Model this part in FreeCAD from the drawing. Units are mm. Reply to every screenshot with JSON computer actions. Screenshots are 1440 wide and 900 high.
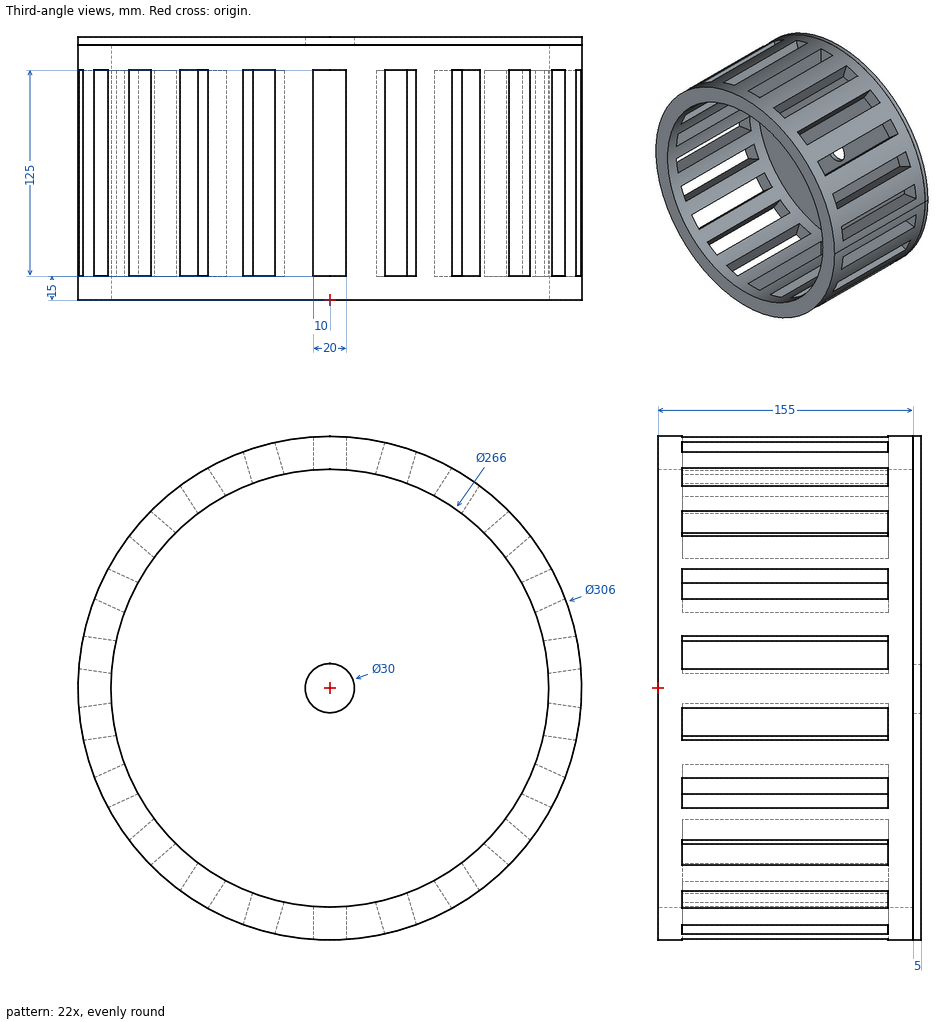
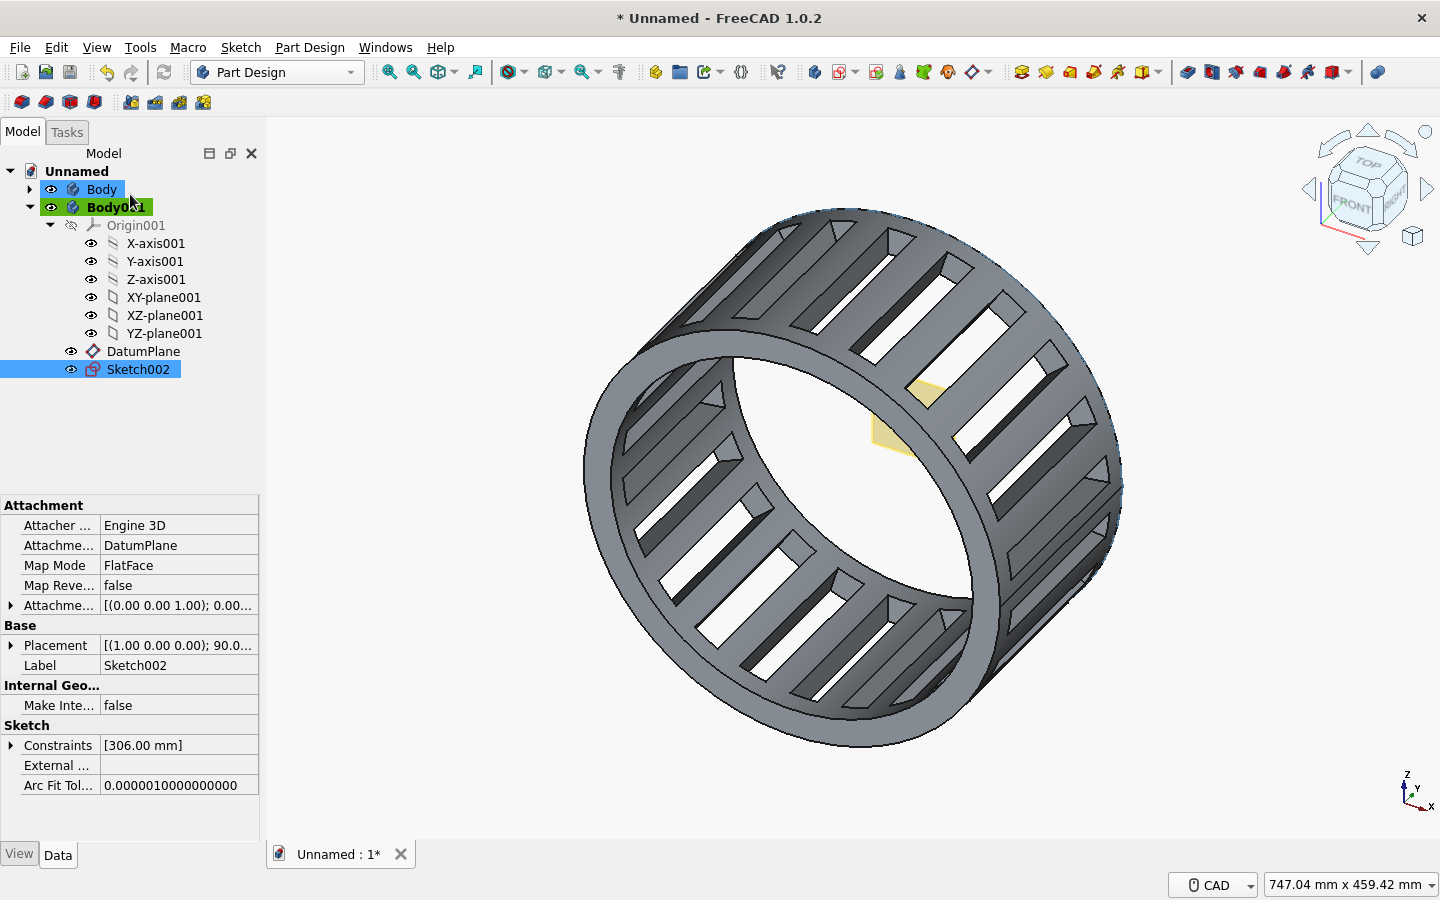
{"action": "left_click", "coordinate": [1022, 72]}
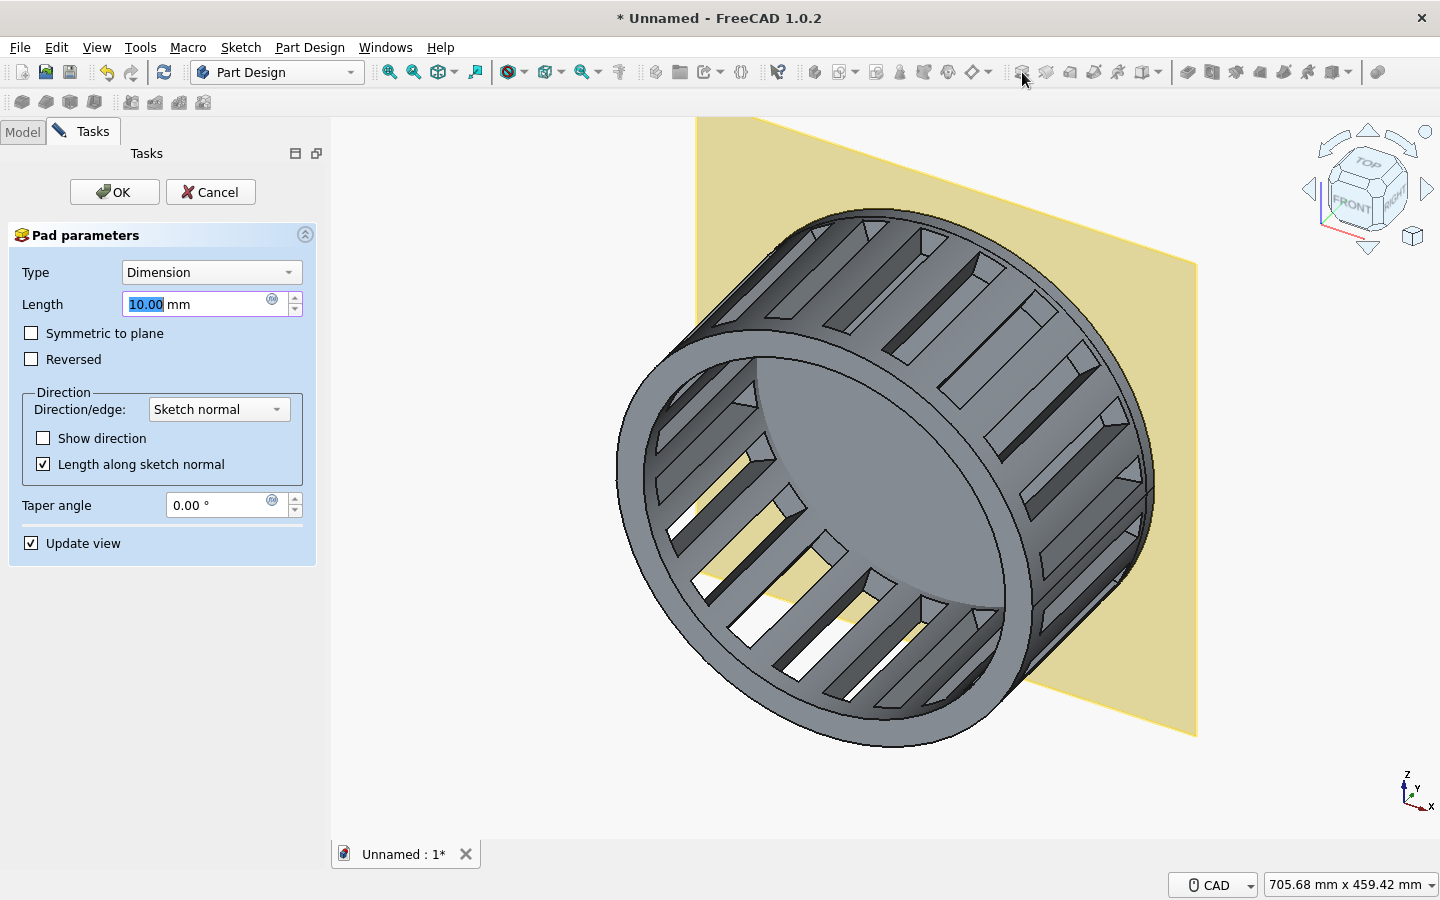
{"action": "type", "text": "5"}
{"action": "key", "text": "Tab"}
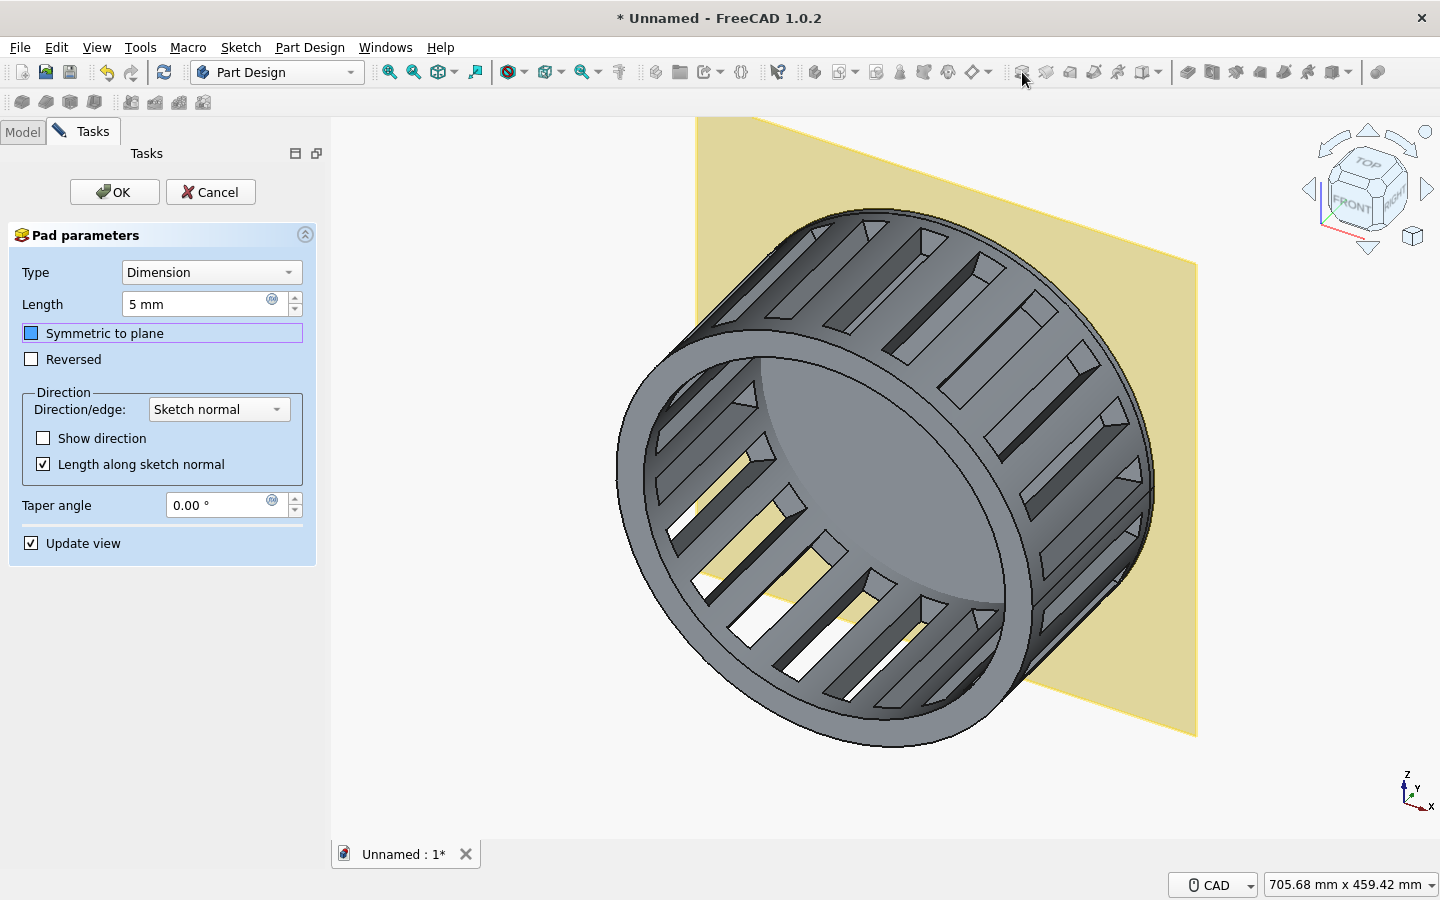
{"action": "left_click", "coordinate": [30, 359]}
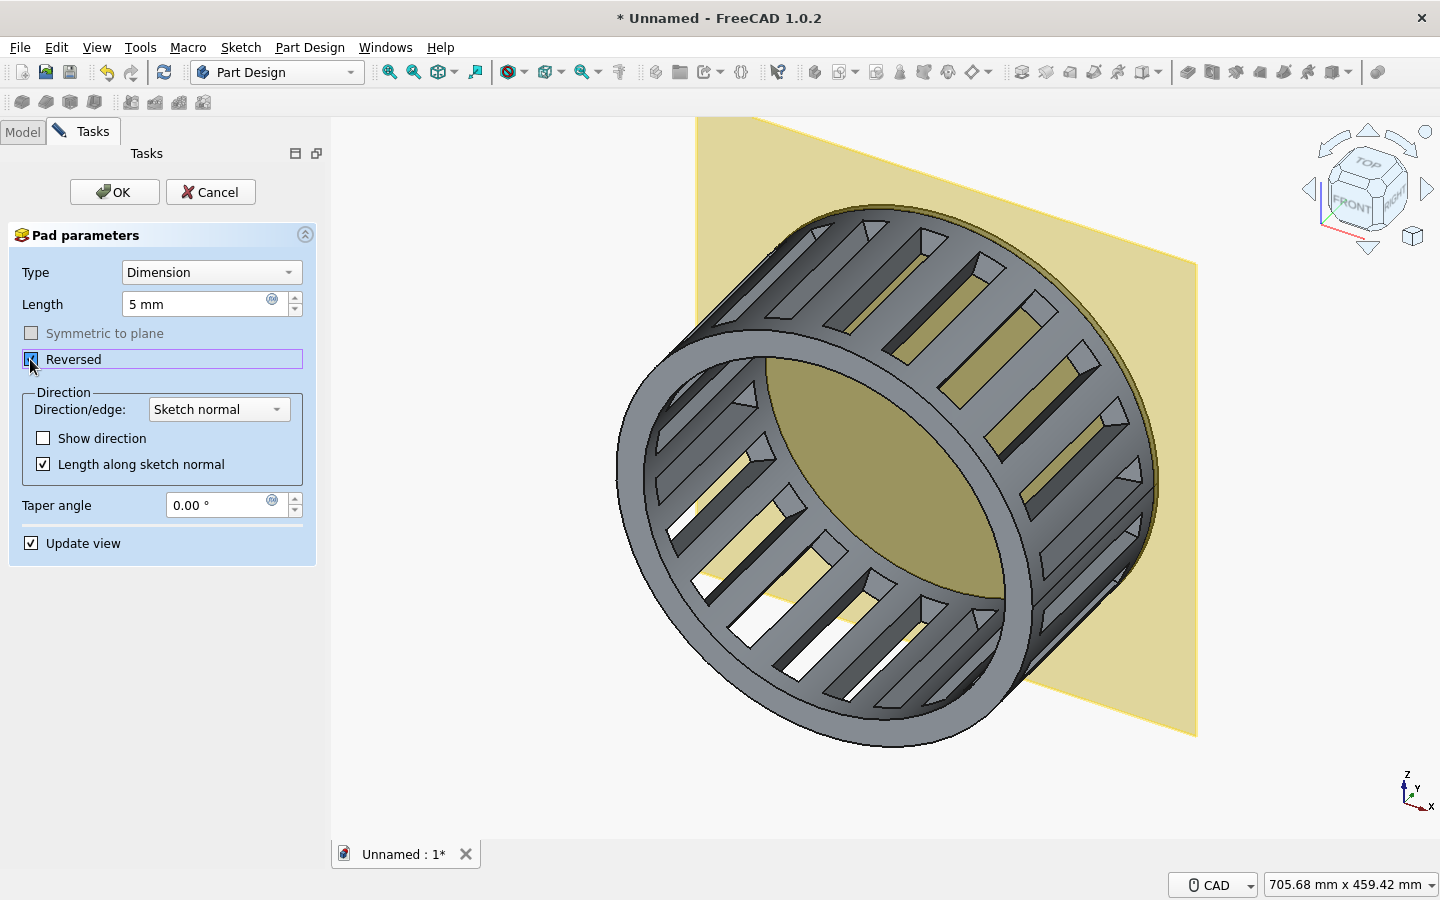
{"action": "left_click", "coordinate": [115, 192]}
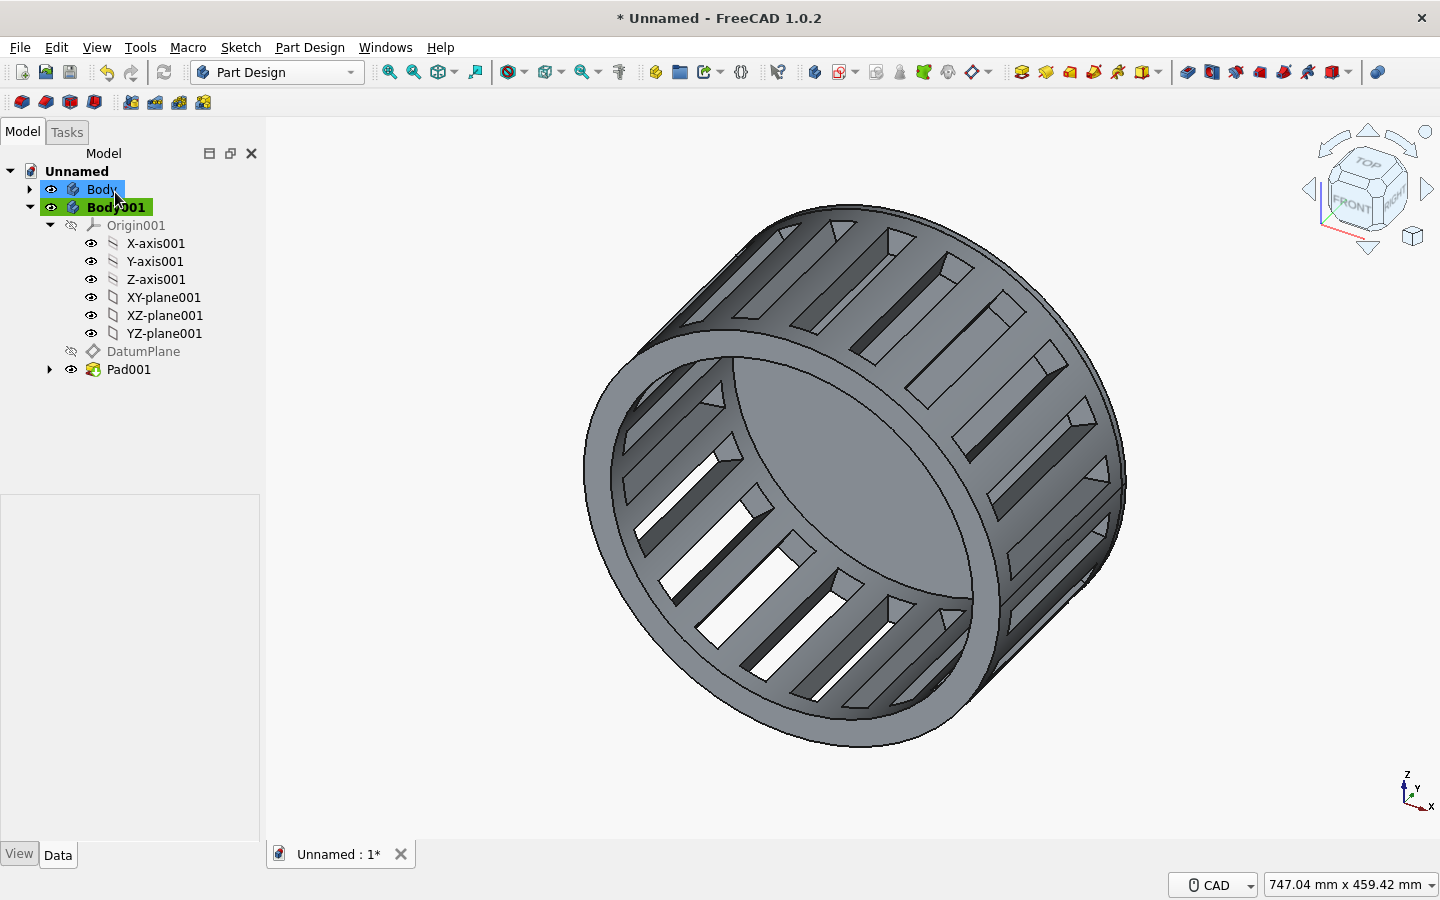
{"action": "key", "text": "4"}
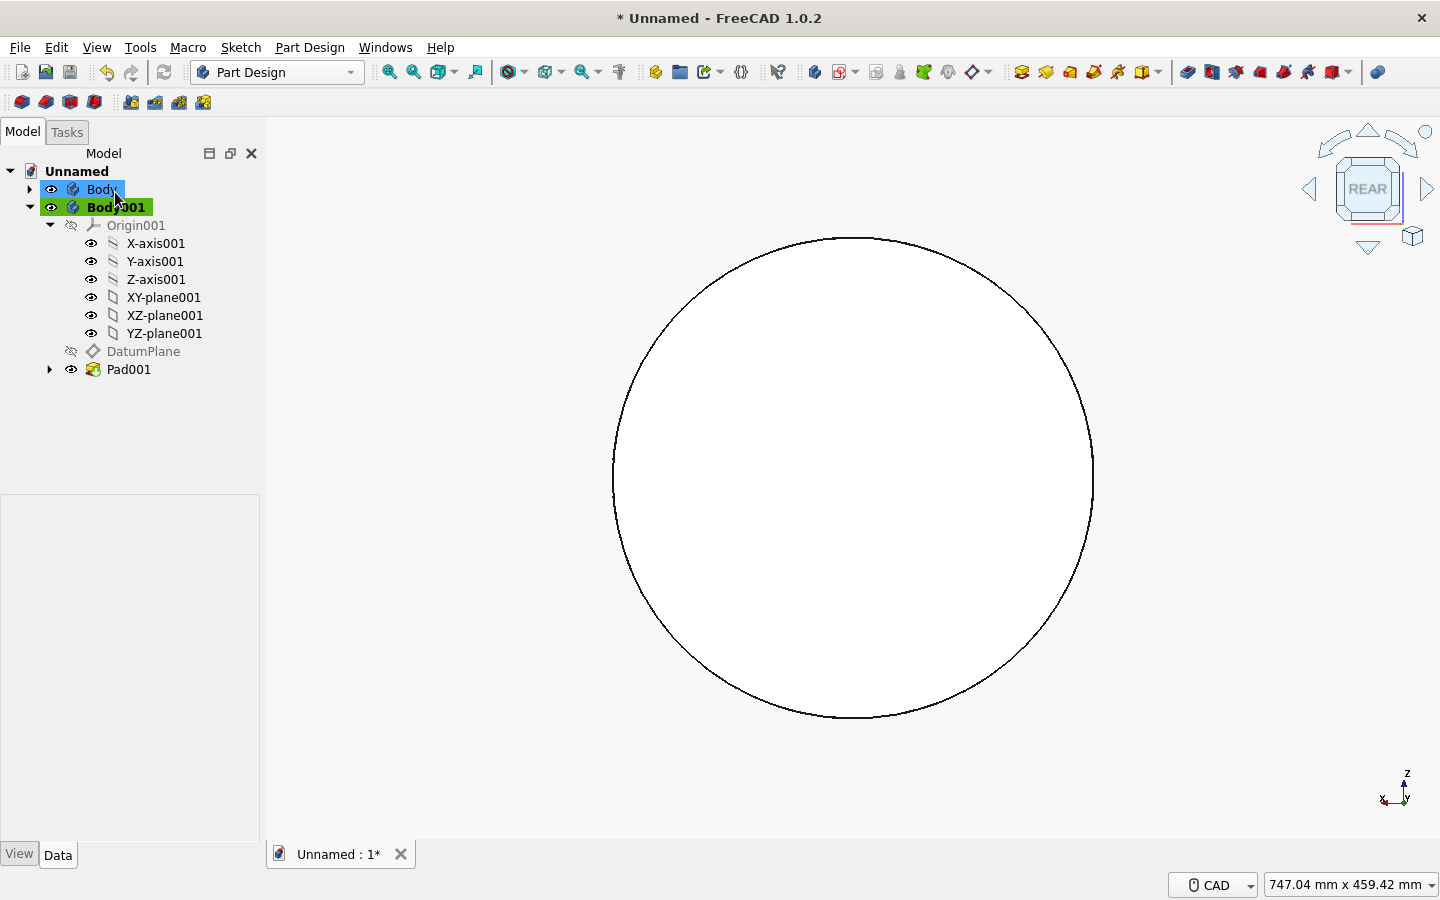
{"action": "left_click", "coordinate": [853, 477]}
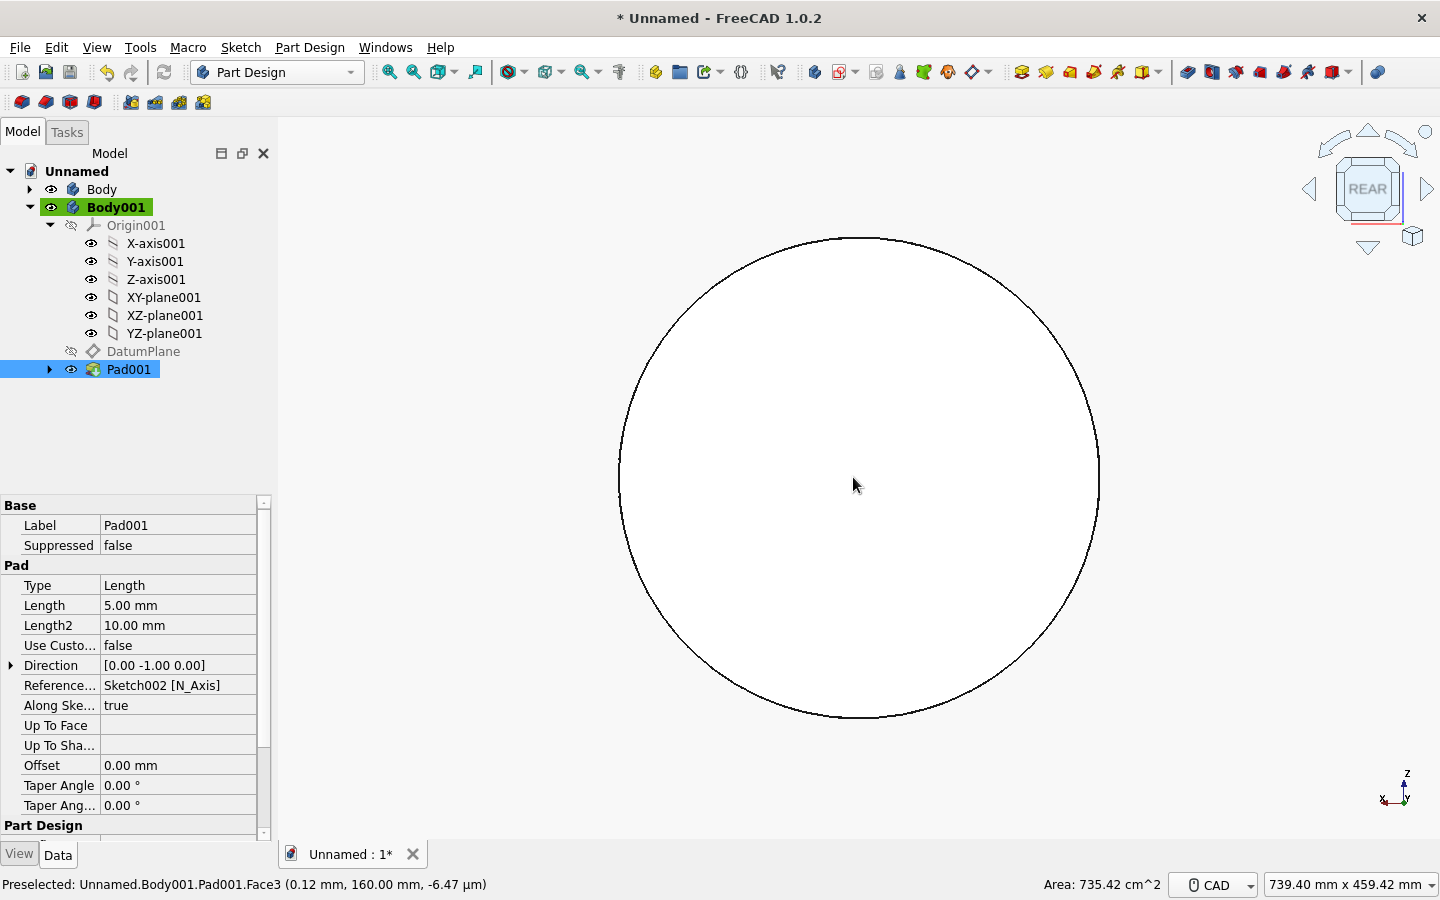
{"action": "left_click", "coordinate": [840, 72]}